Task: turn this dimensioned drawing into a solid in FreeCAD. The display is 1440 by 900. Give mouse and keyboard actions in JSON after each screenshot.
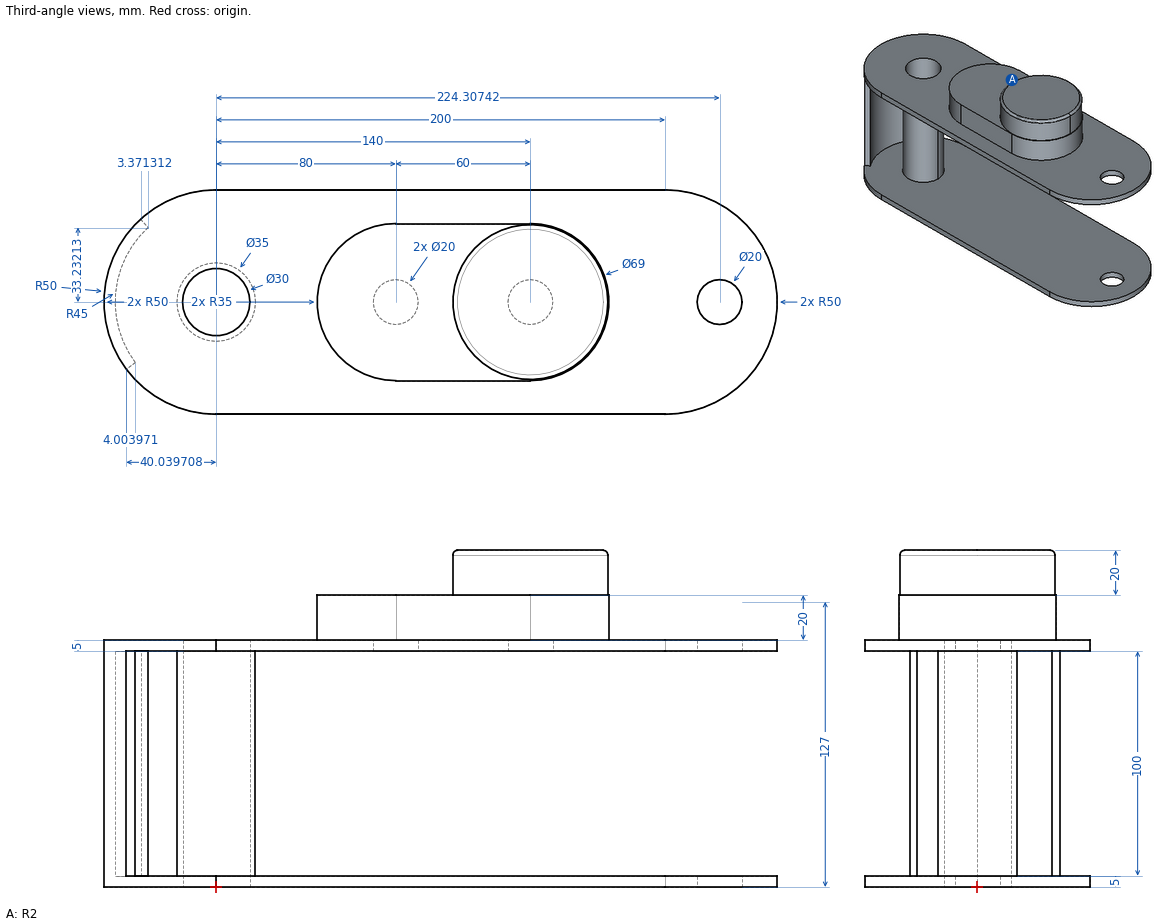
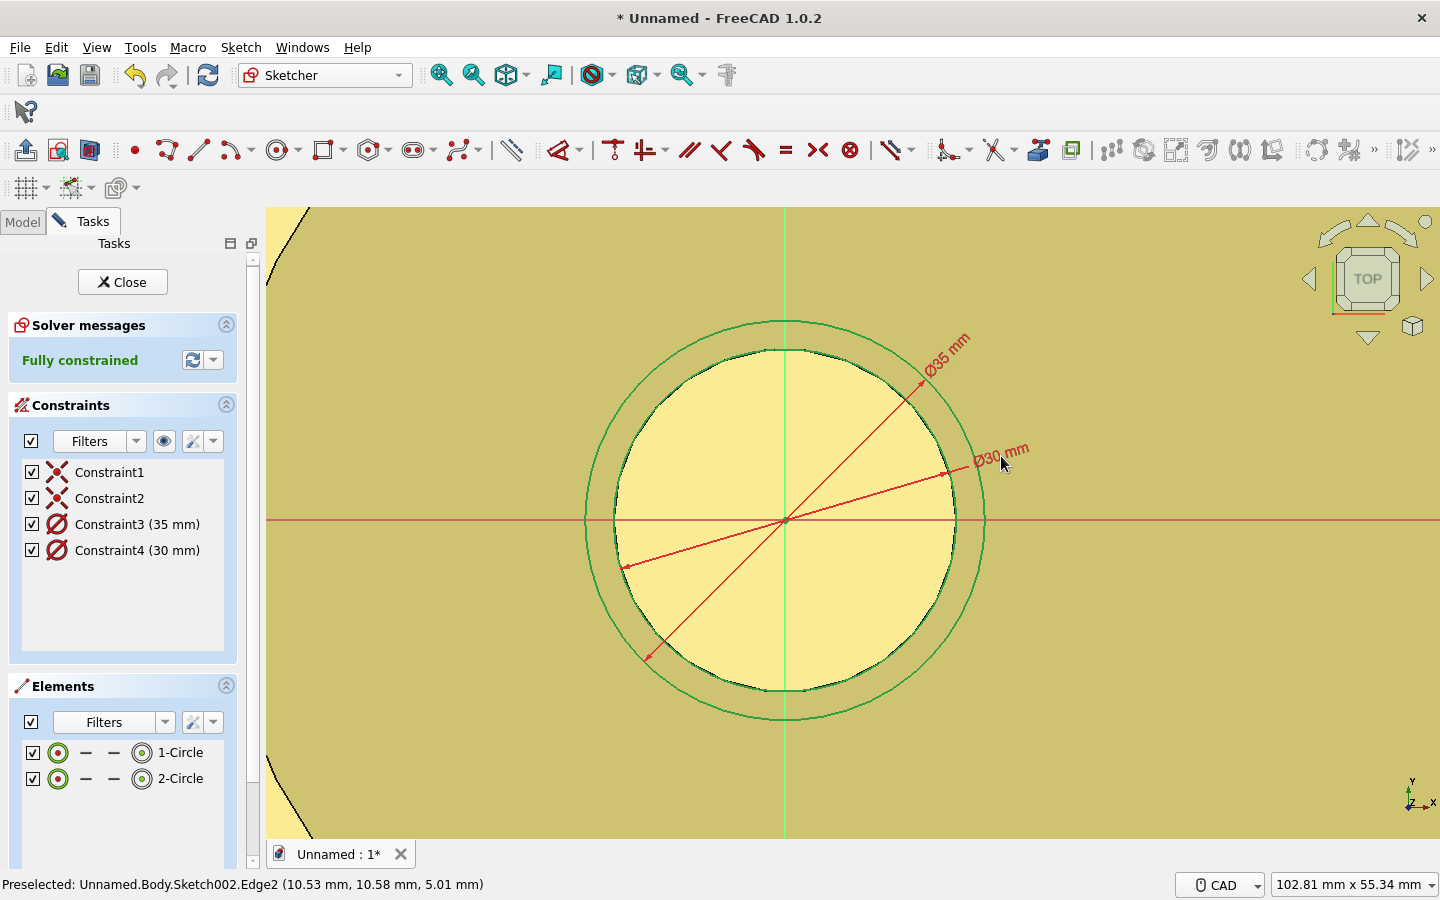
{"action": "left_click", "coordinate": [123, 282]}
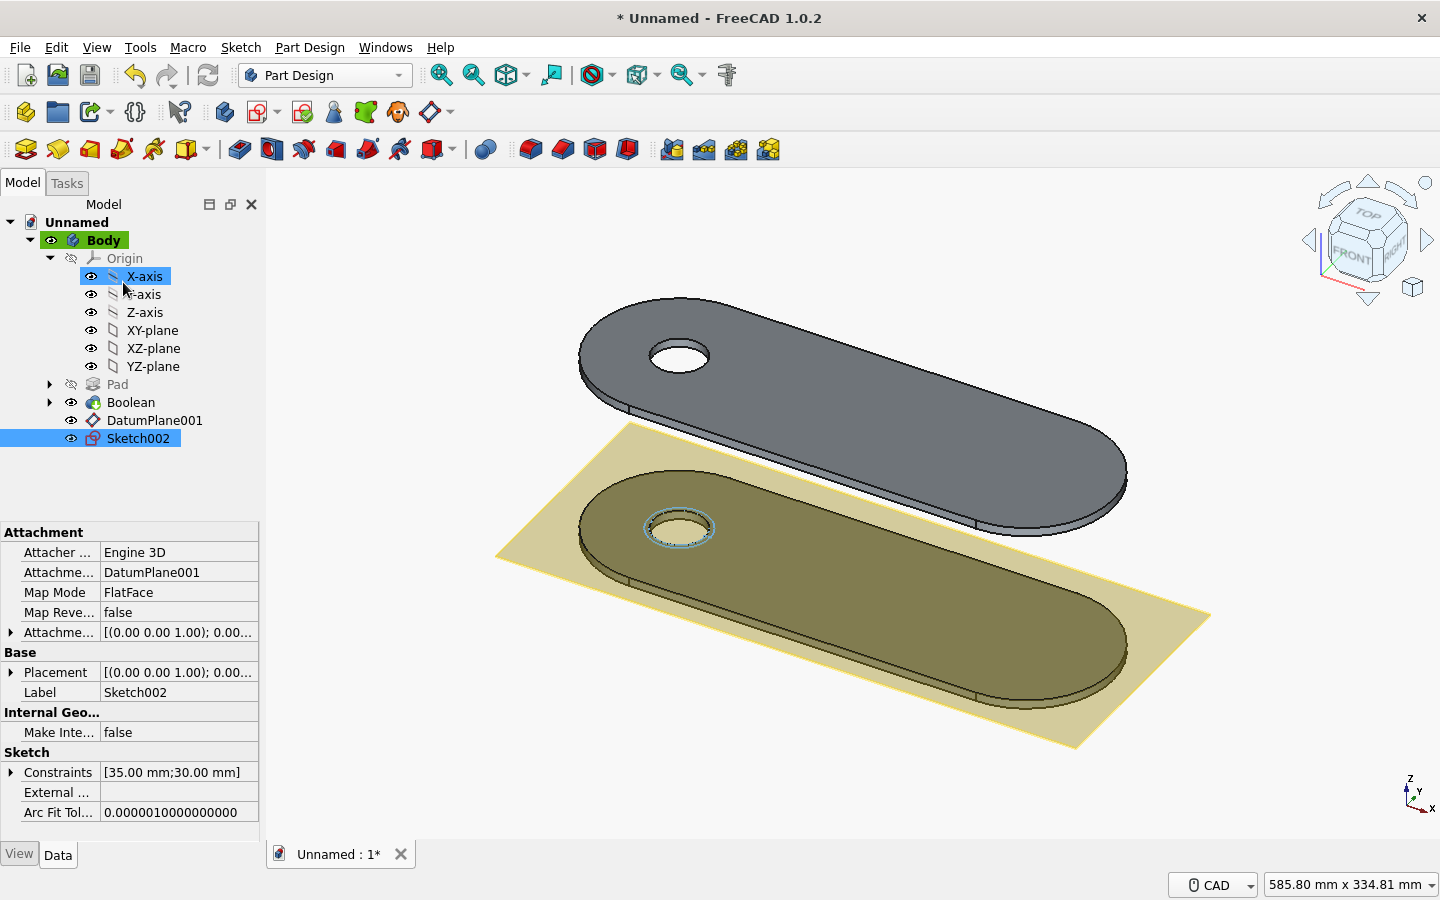
{"action": "left_click", "coordinate": [26, 150]}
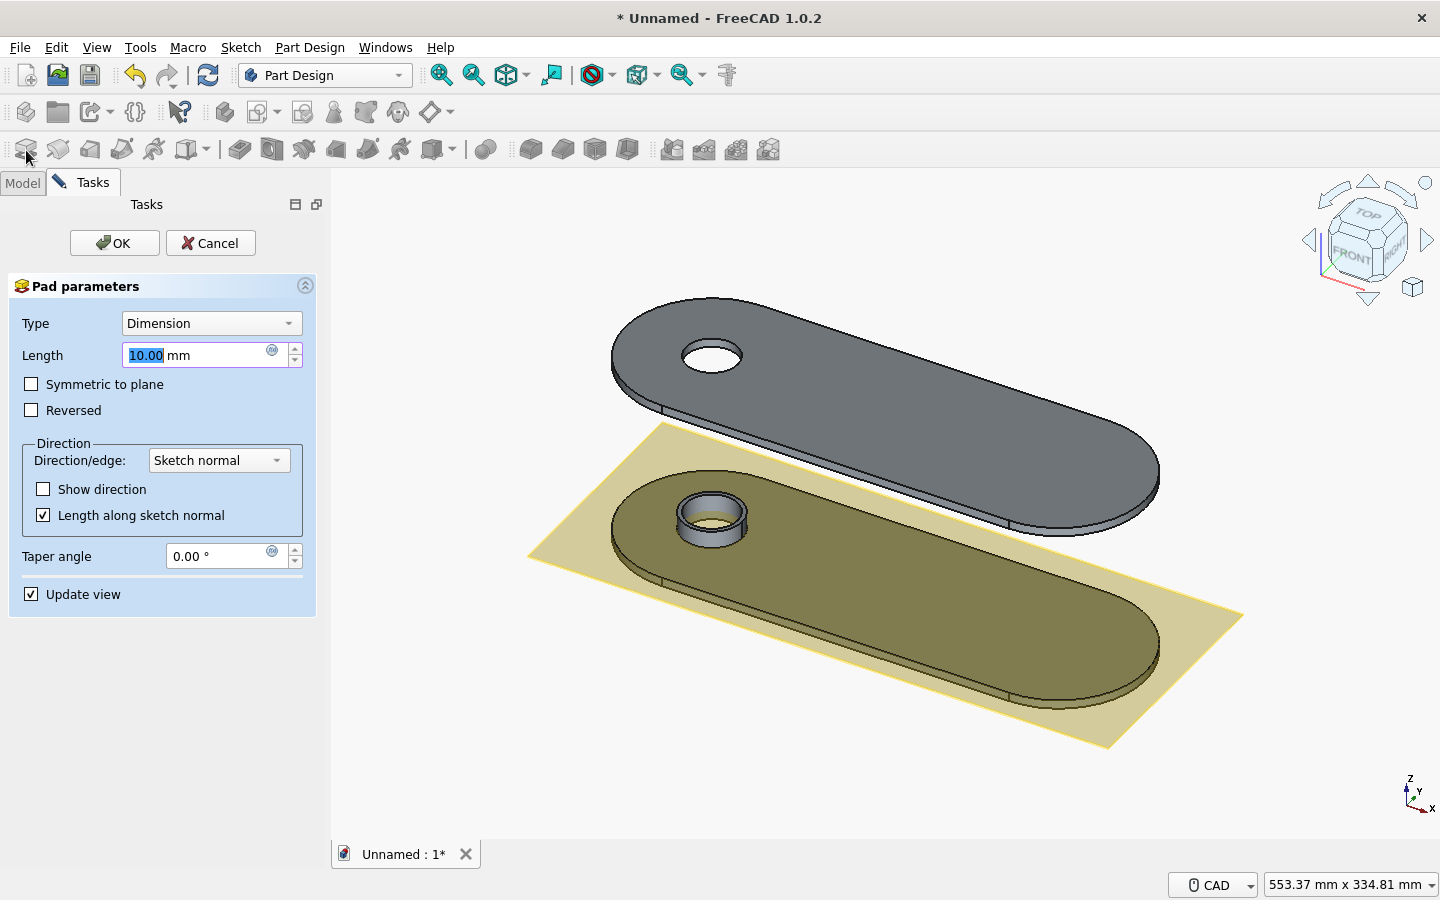
{"action": "type", "text": "100"}
{"action": "key", "text": "Tab"}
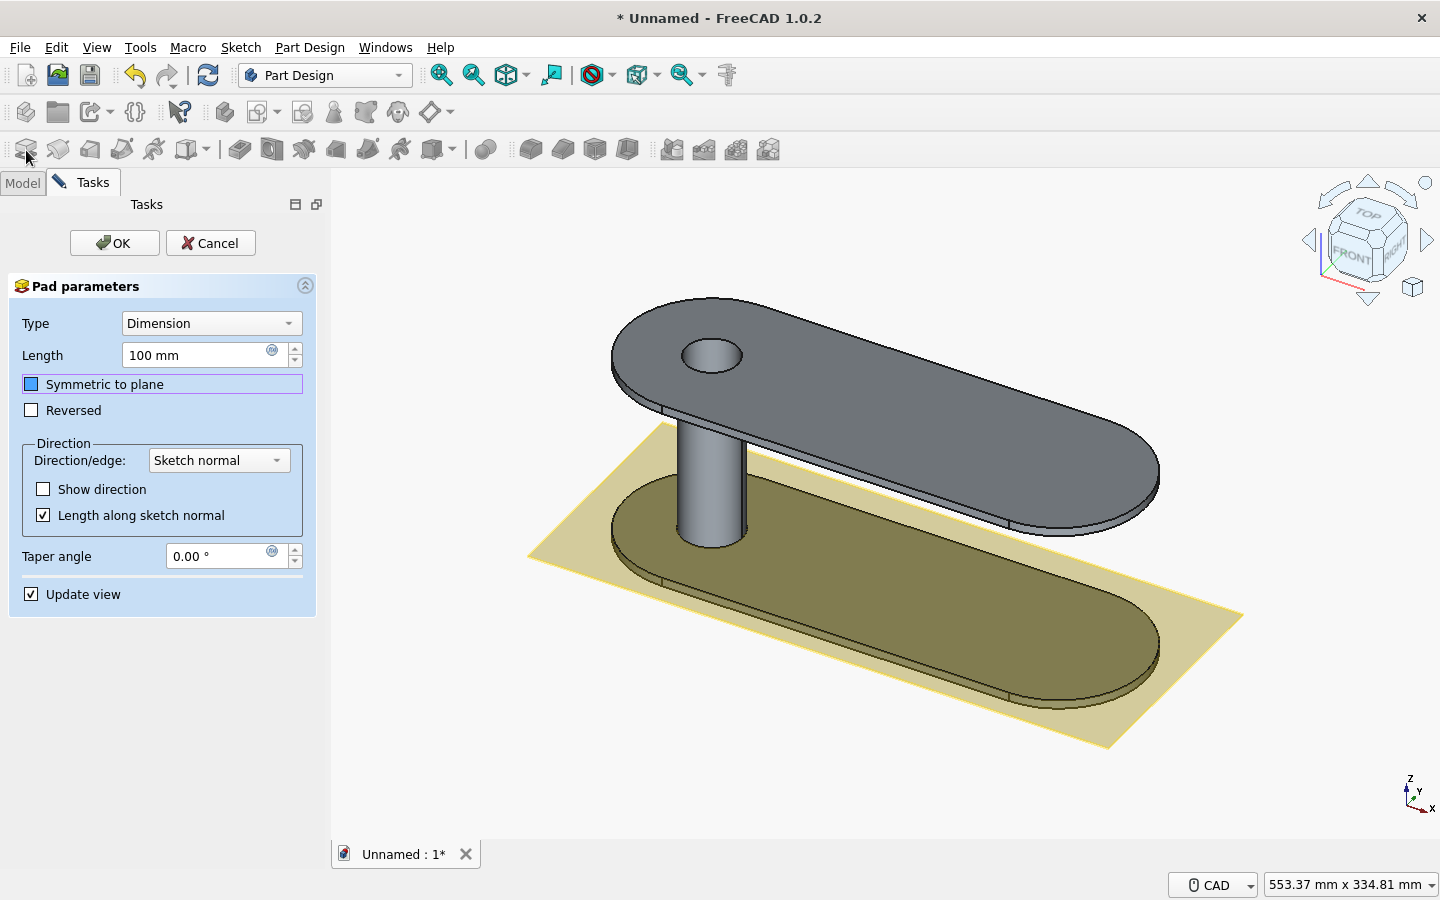
{"action": "left_click", "coordinate": [115, 243]}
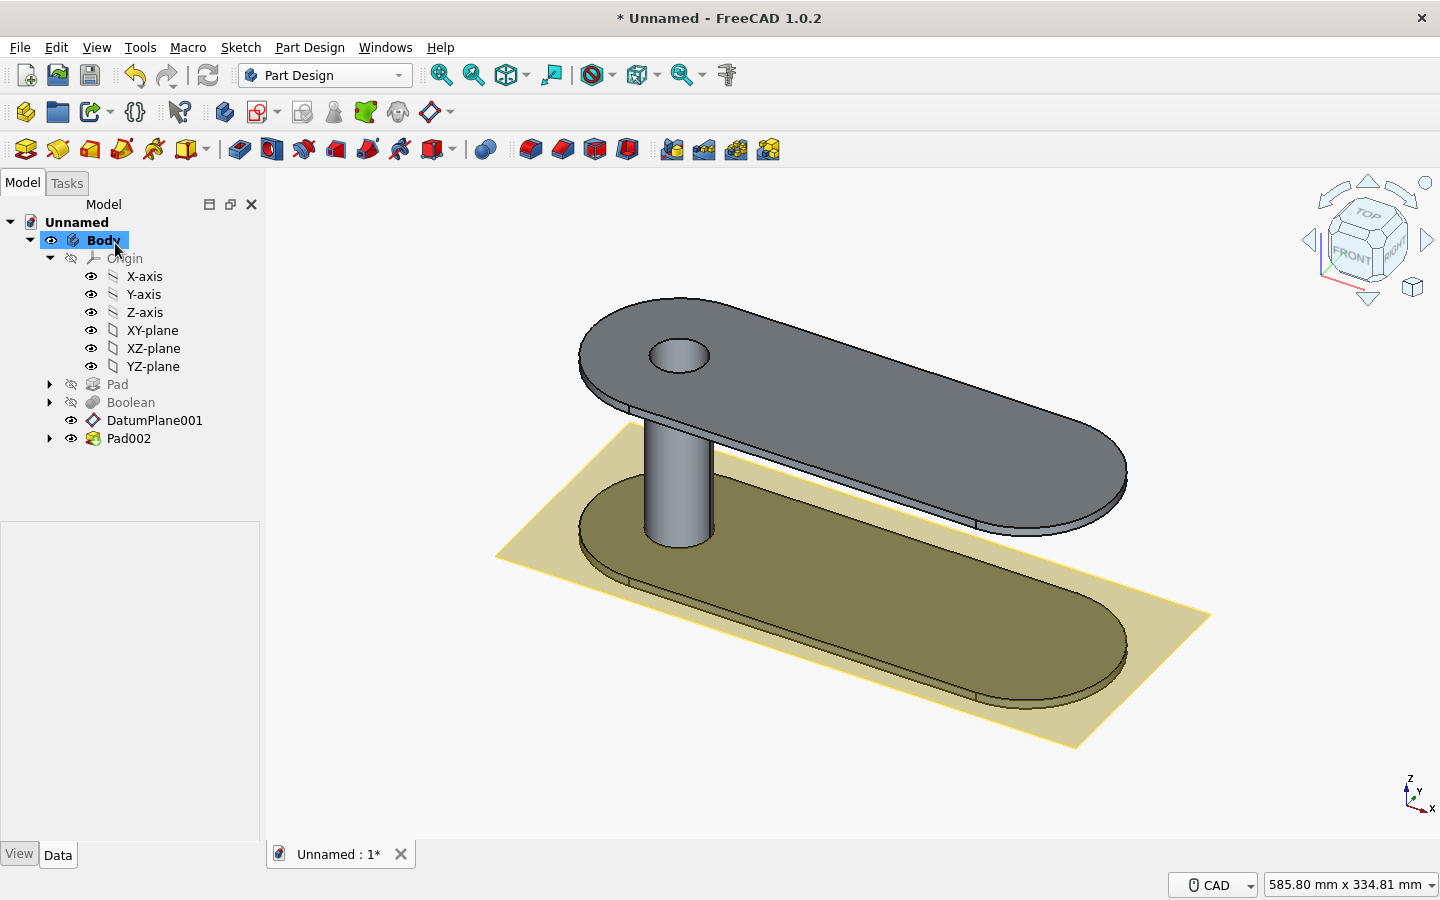
{"action": "left_click", "coordinate": [116, 420]}
{"action": "key", "text": "space"}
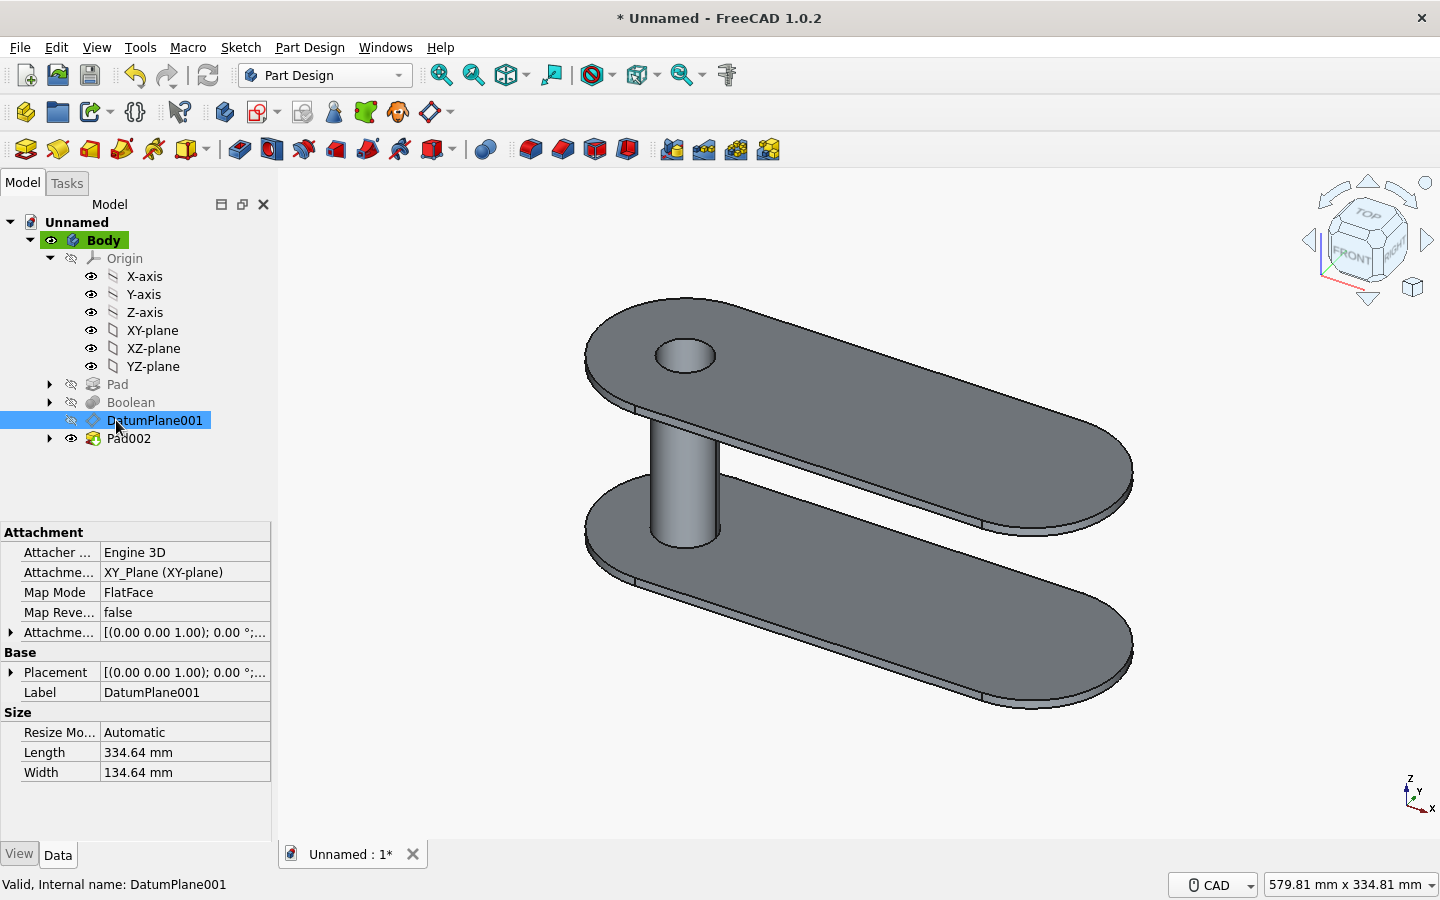
{"action": "left_click", "coordinate": [136, 330]}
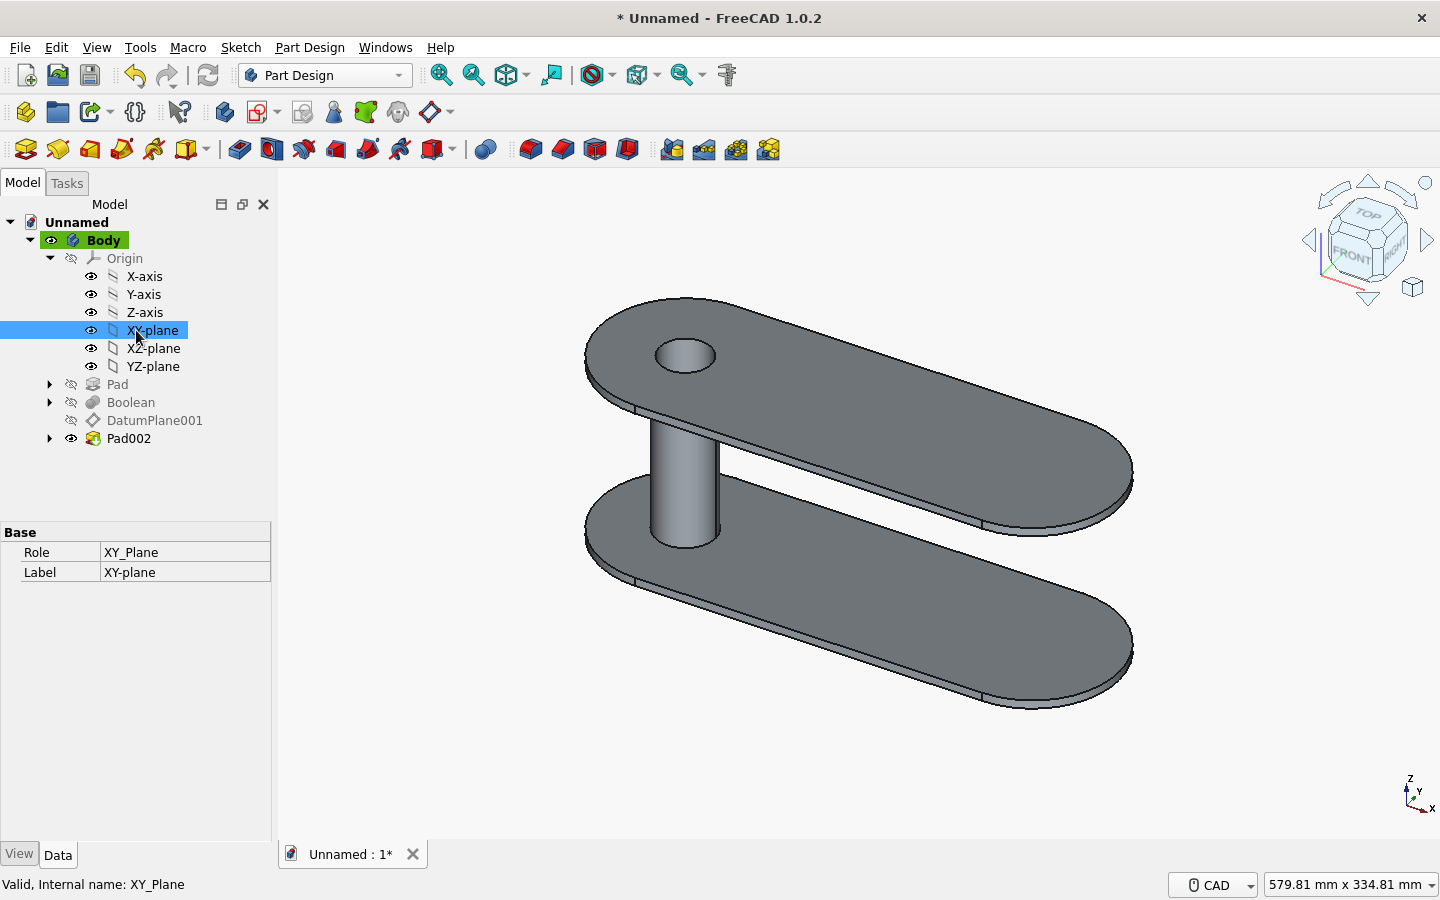
{"action": "left_click", "coordinate": [430, 112]}